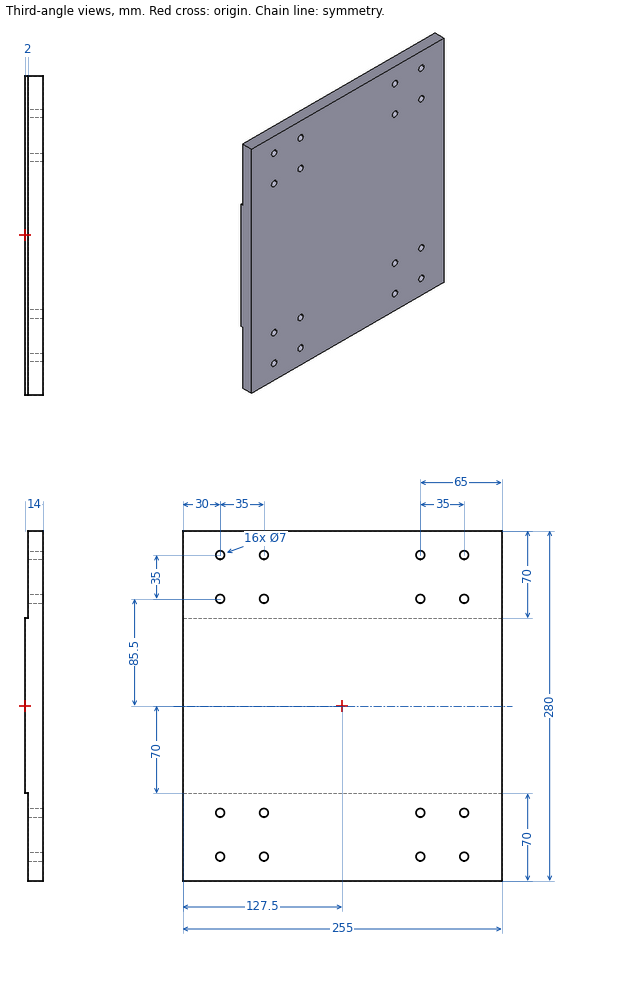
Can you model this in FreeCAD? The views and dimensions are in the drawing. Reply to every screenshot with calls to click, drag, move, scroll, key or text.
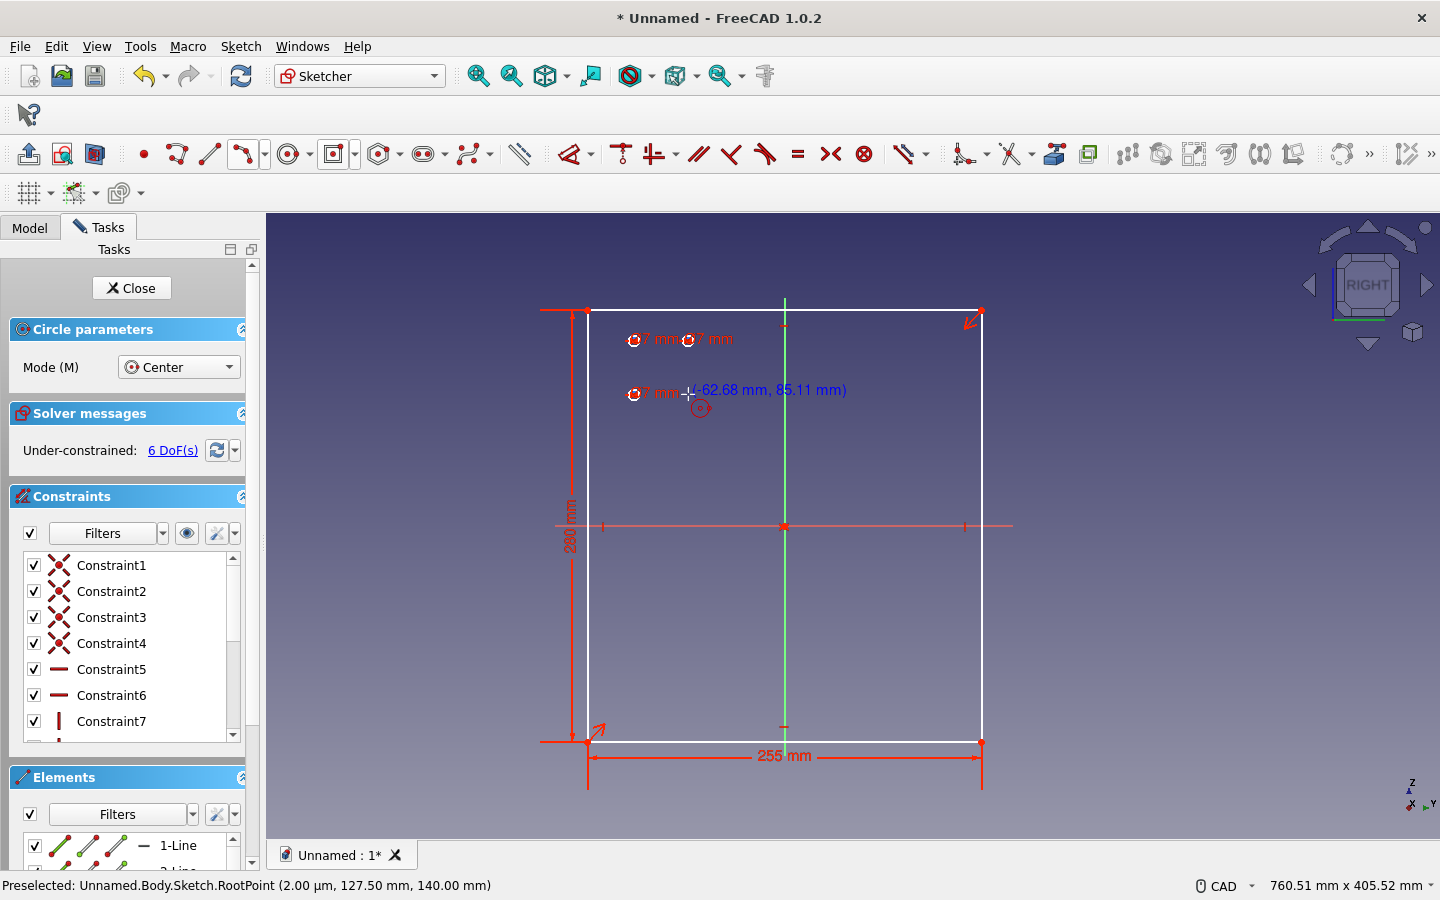
click(688, 394)
move(692, 391)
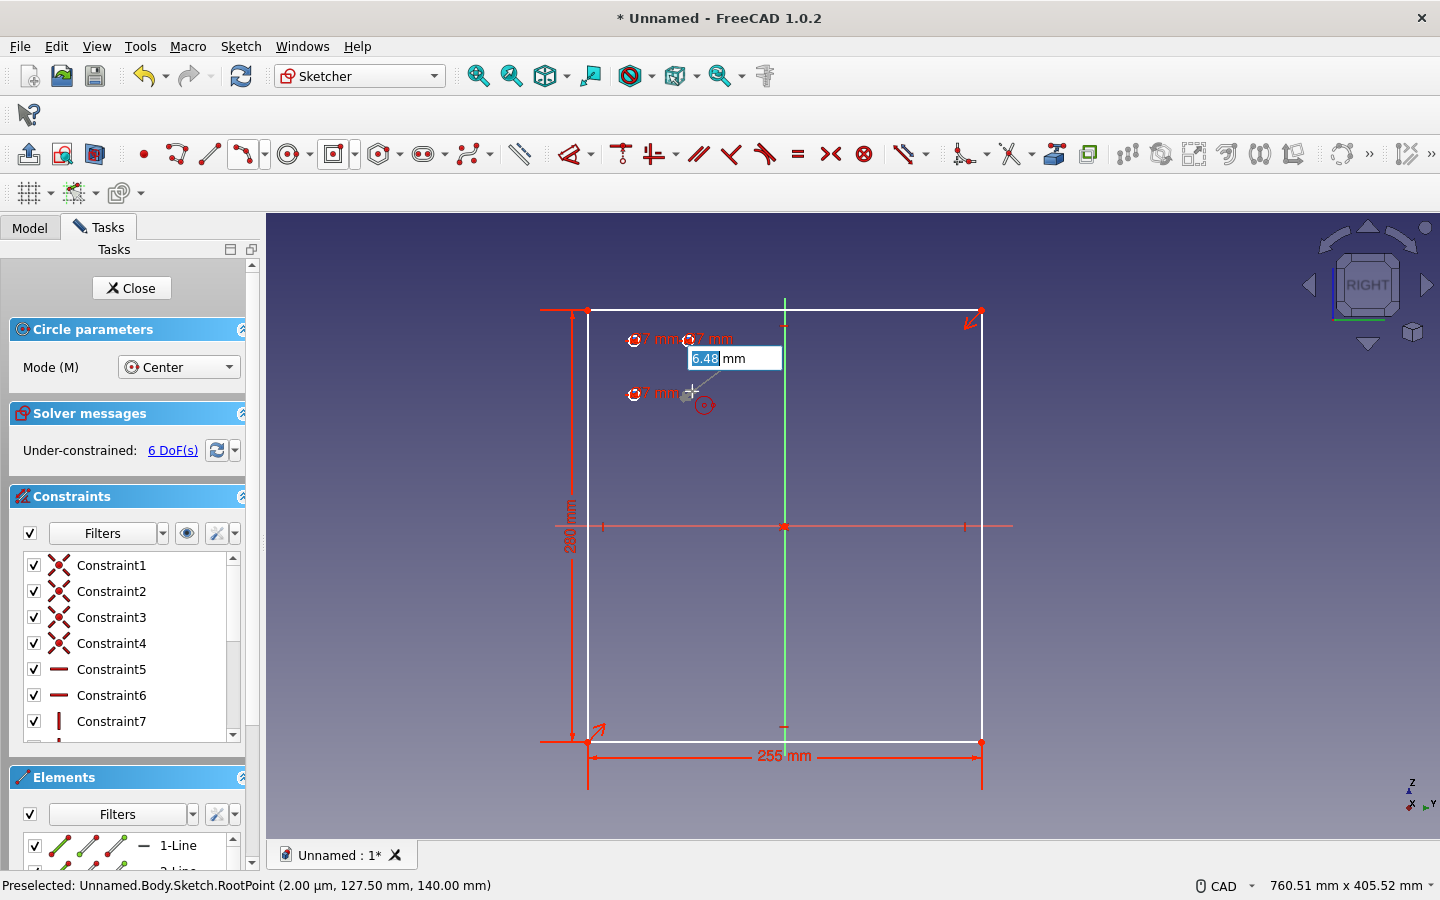
text(7)
key(Return)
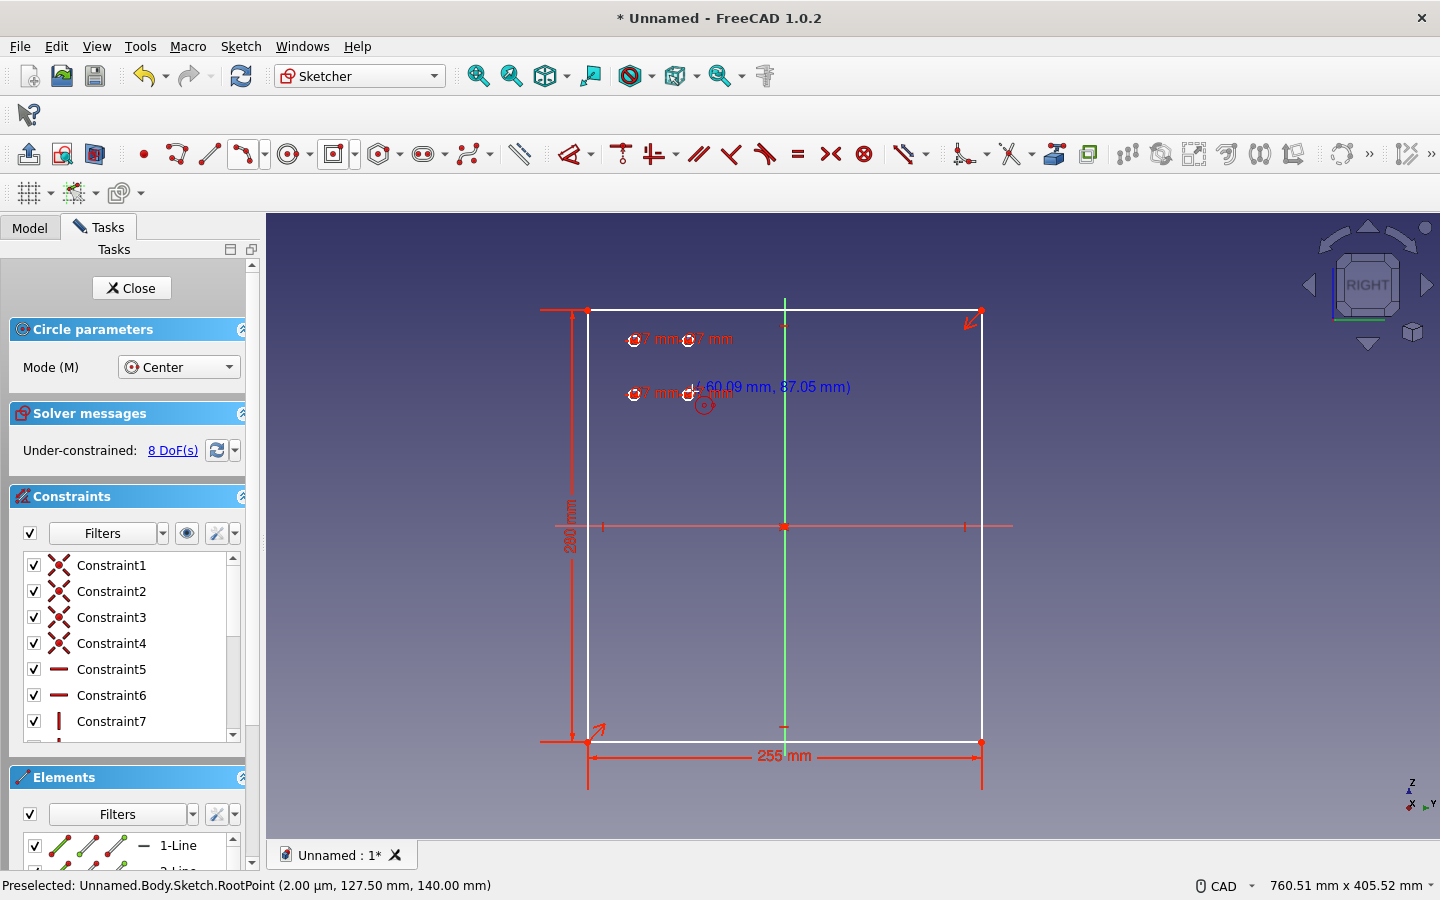
scroll(634, 658, up, 8)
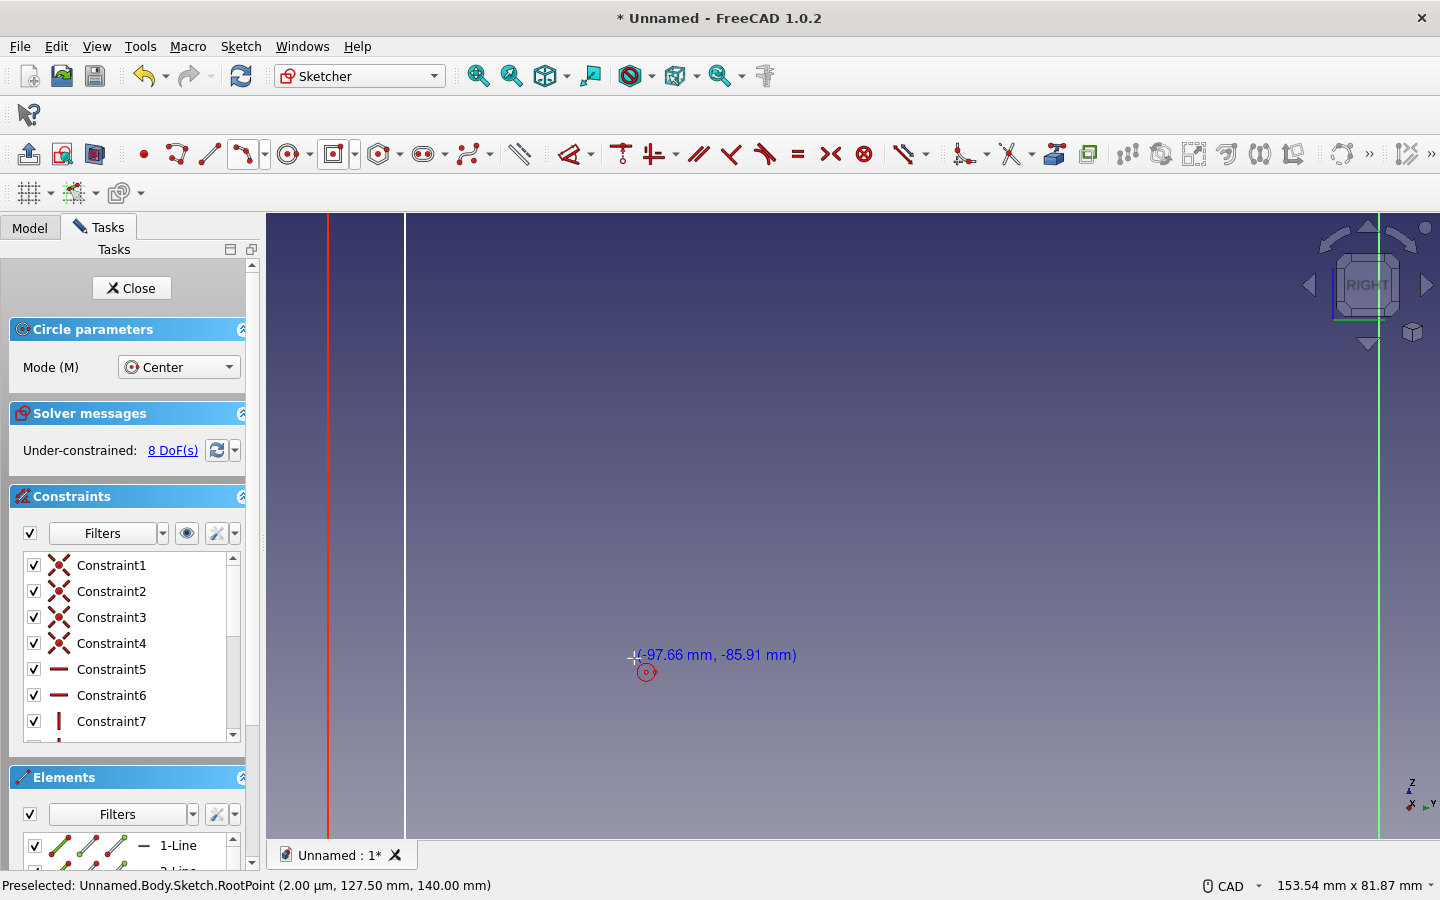
scroll(634, 658, down, 8)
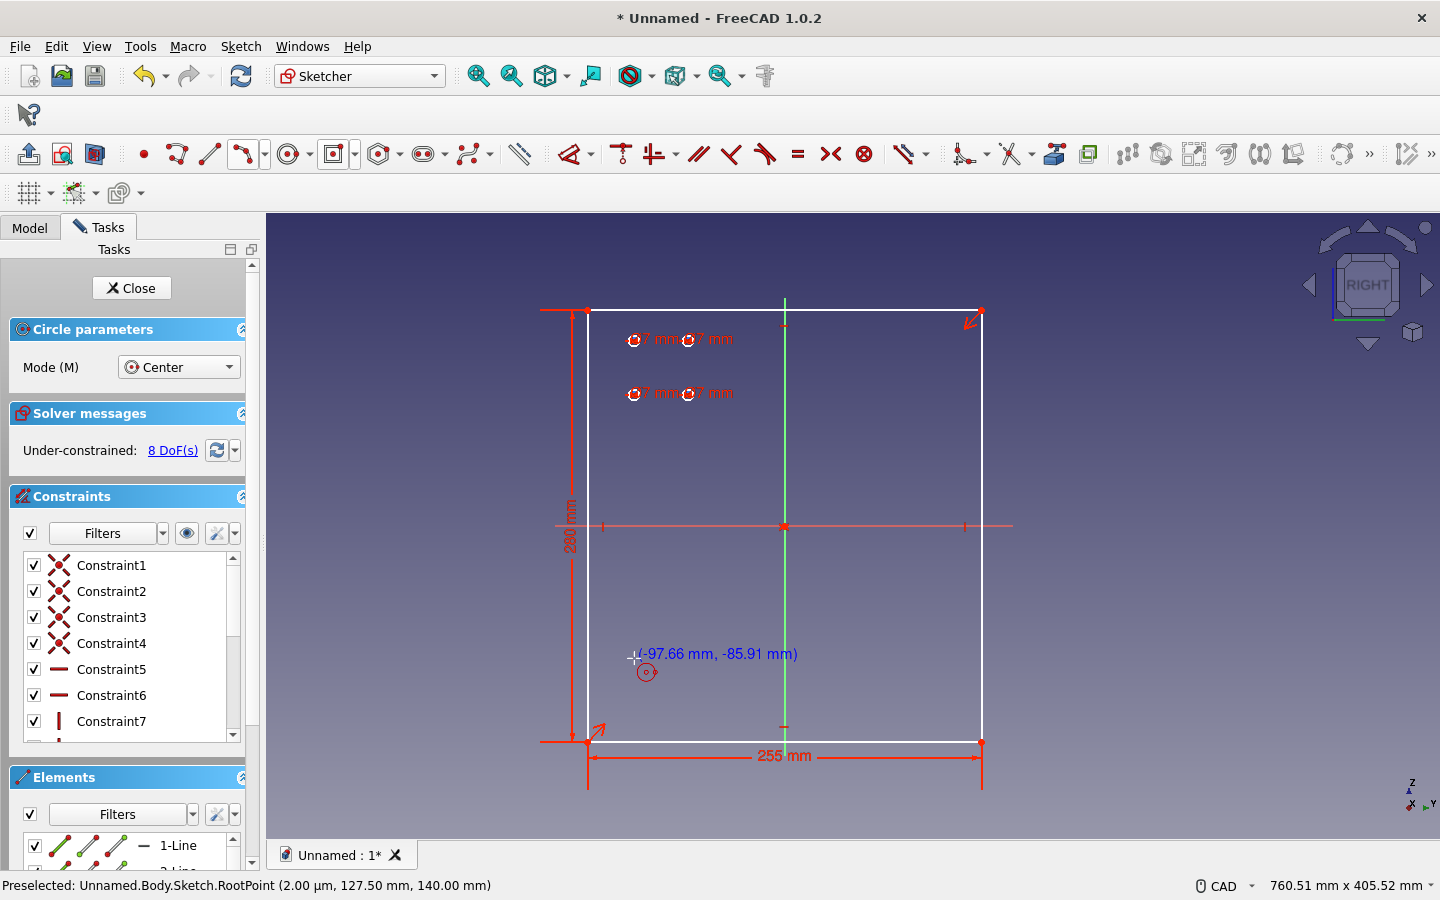
click(634, 658)
move(638, 655)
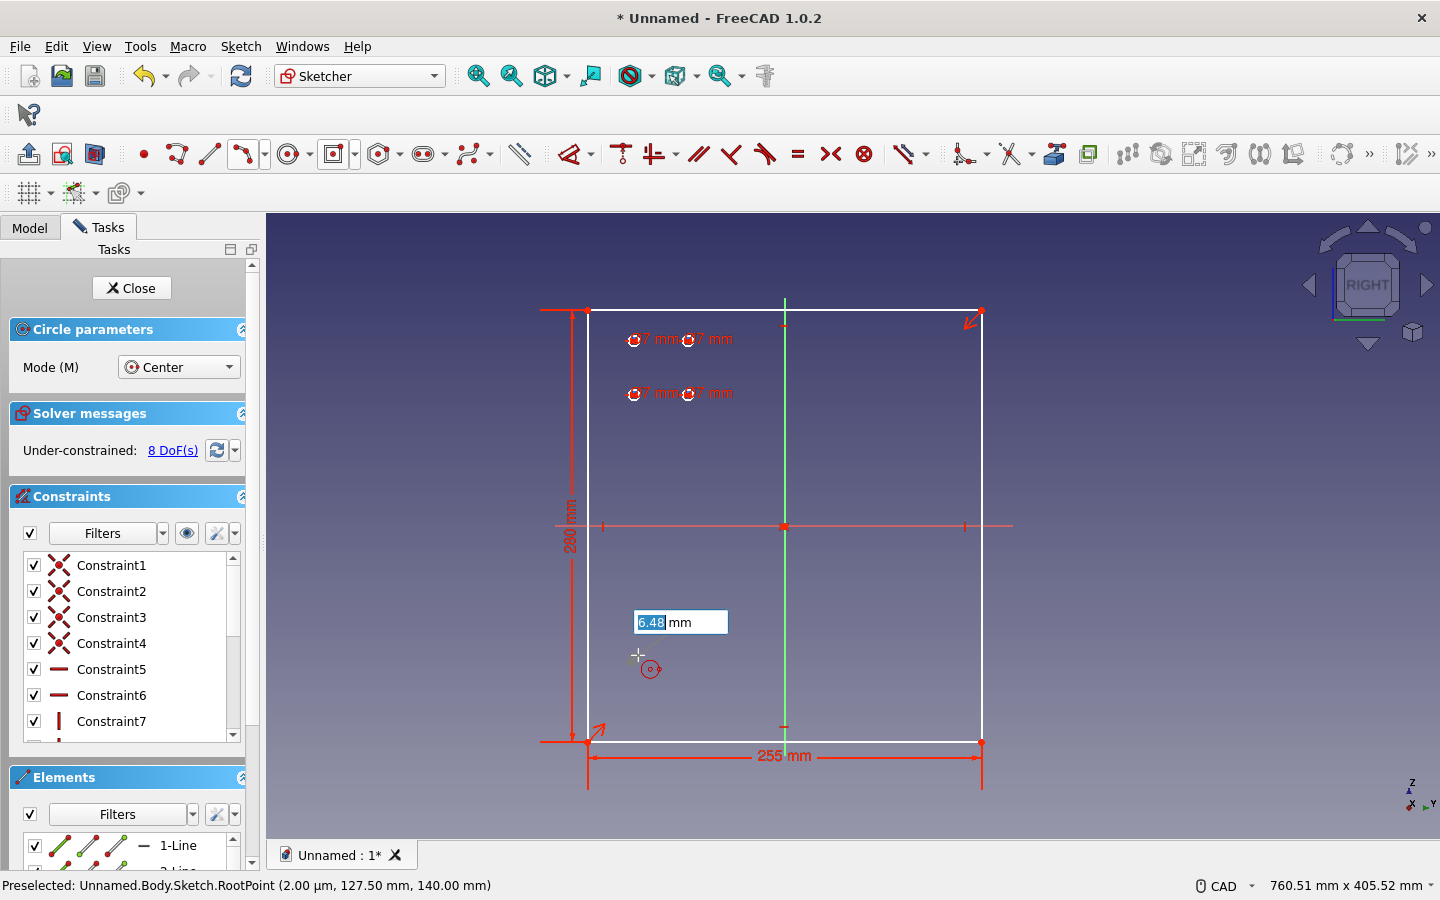
text(7)
key(Return)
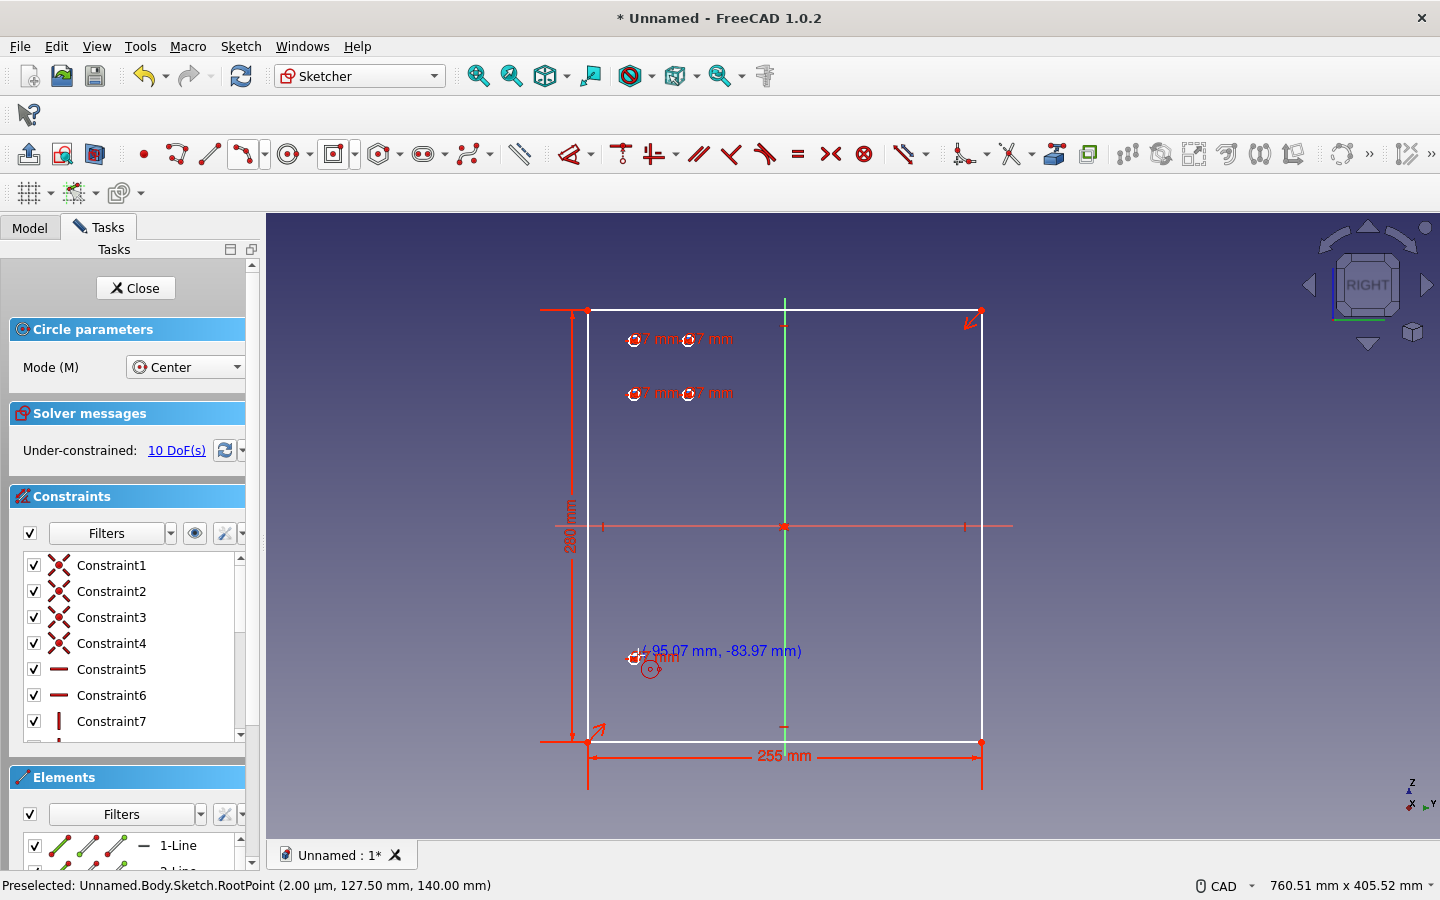
scroll(634, 712, up, 8)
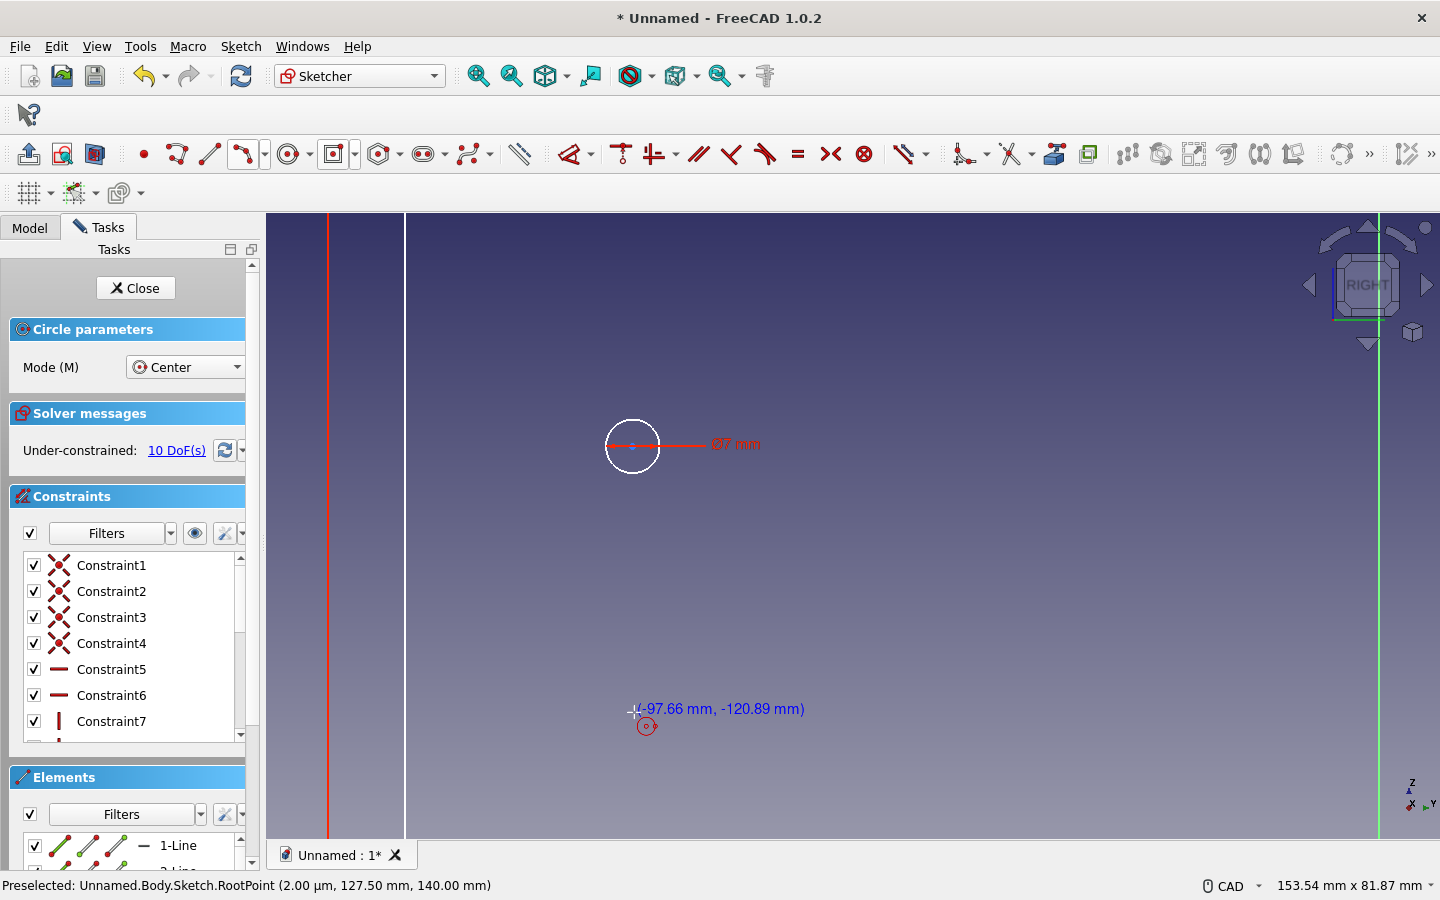
scroll(634, 712, down, 8)